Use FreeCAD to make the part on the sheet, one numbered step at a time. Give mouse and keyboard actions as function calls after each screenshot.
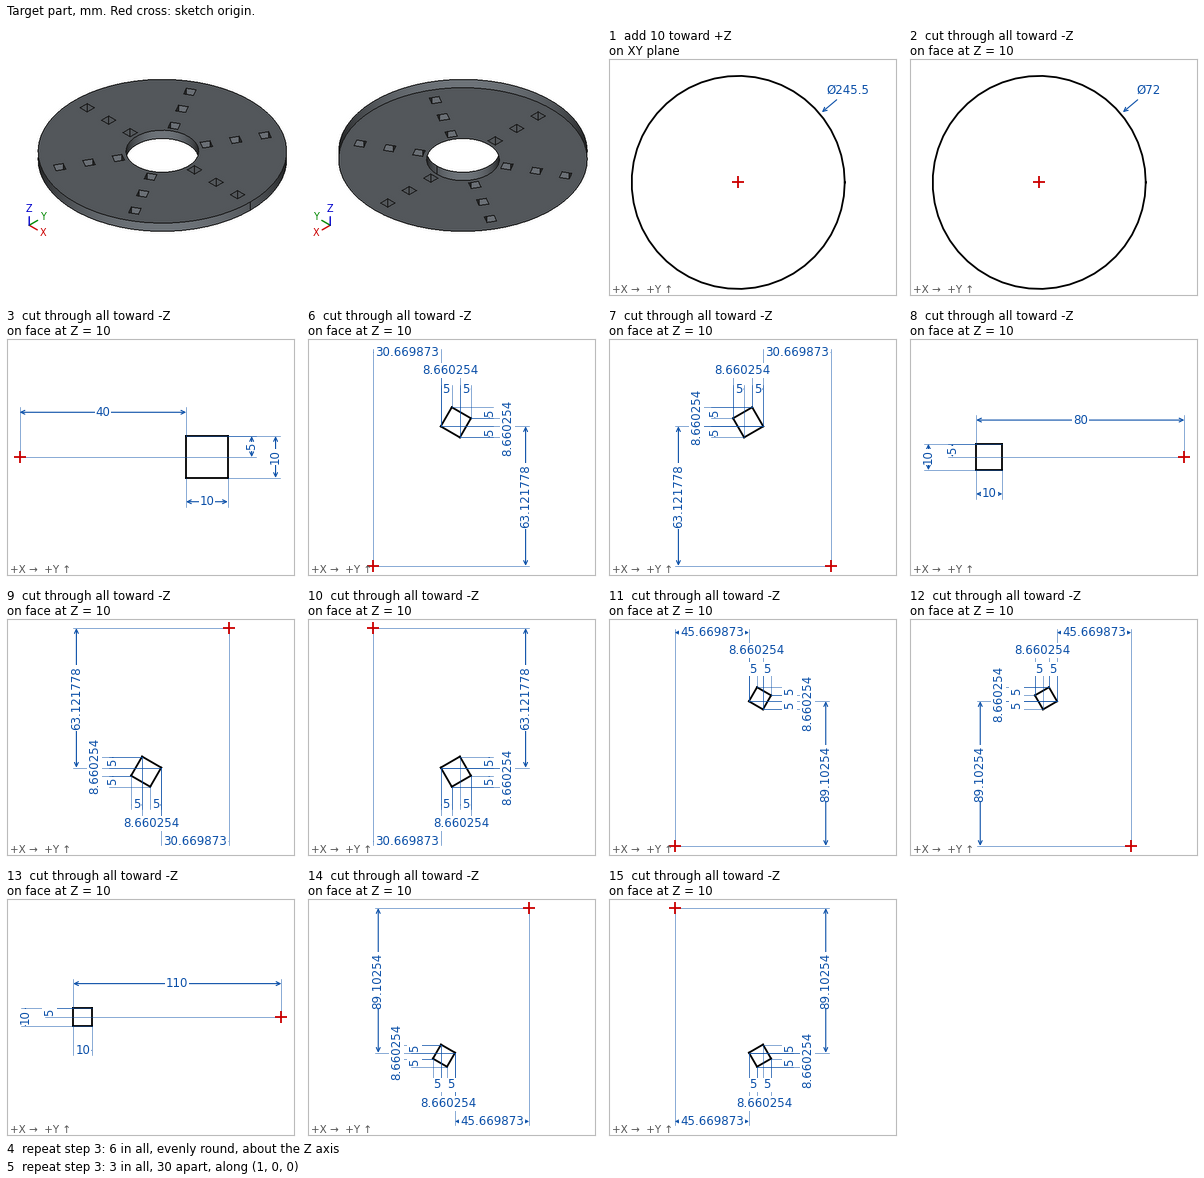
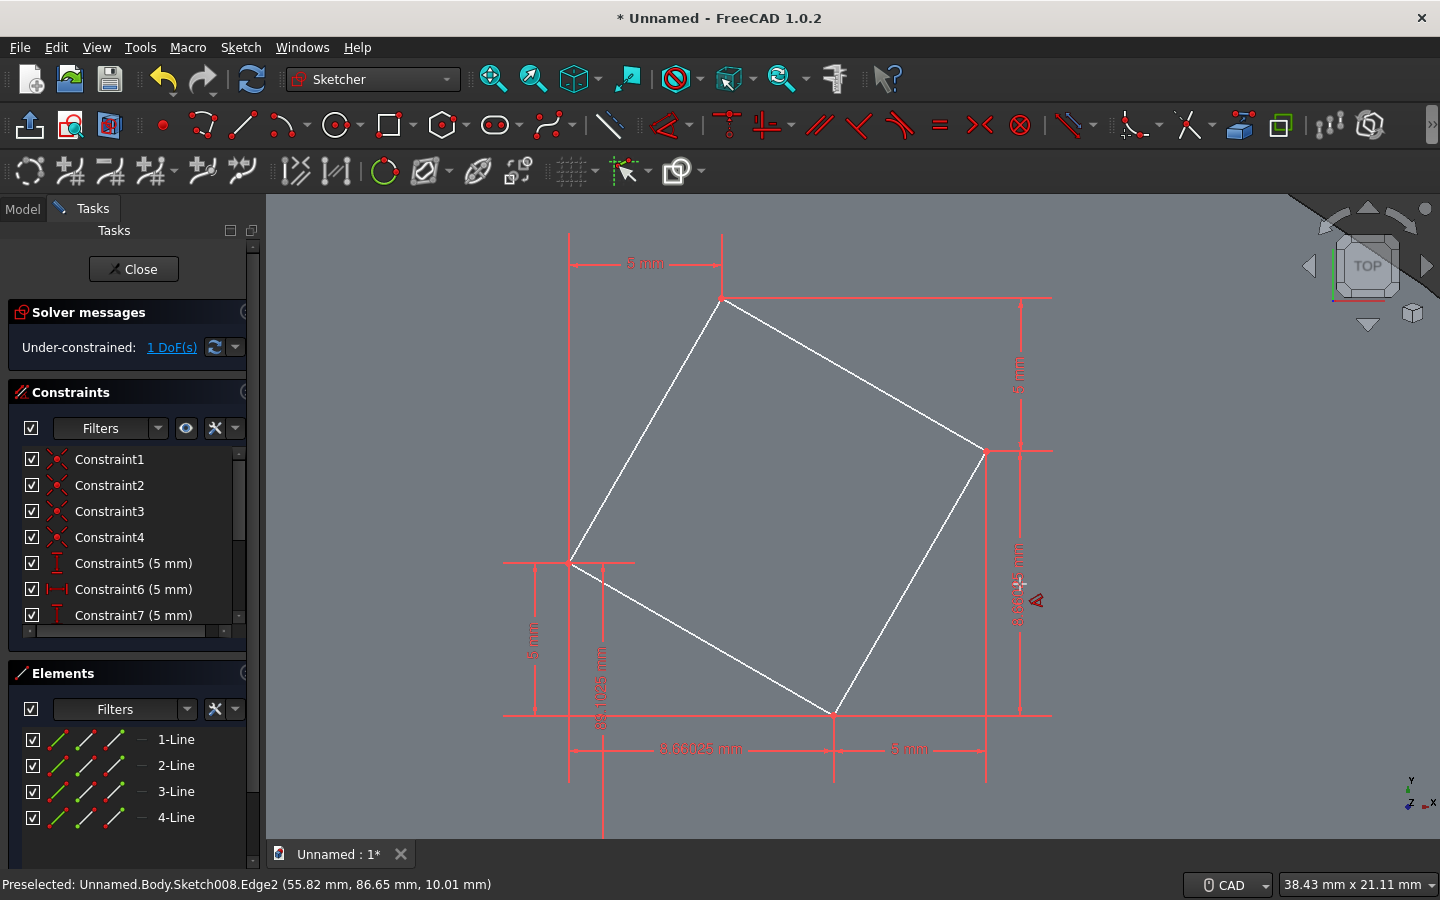
click(569, 563)
click(431, 529)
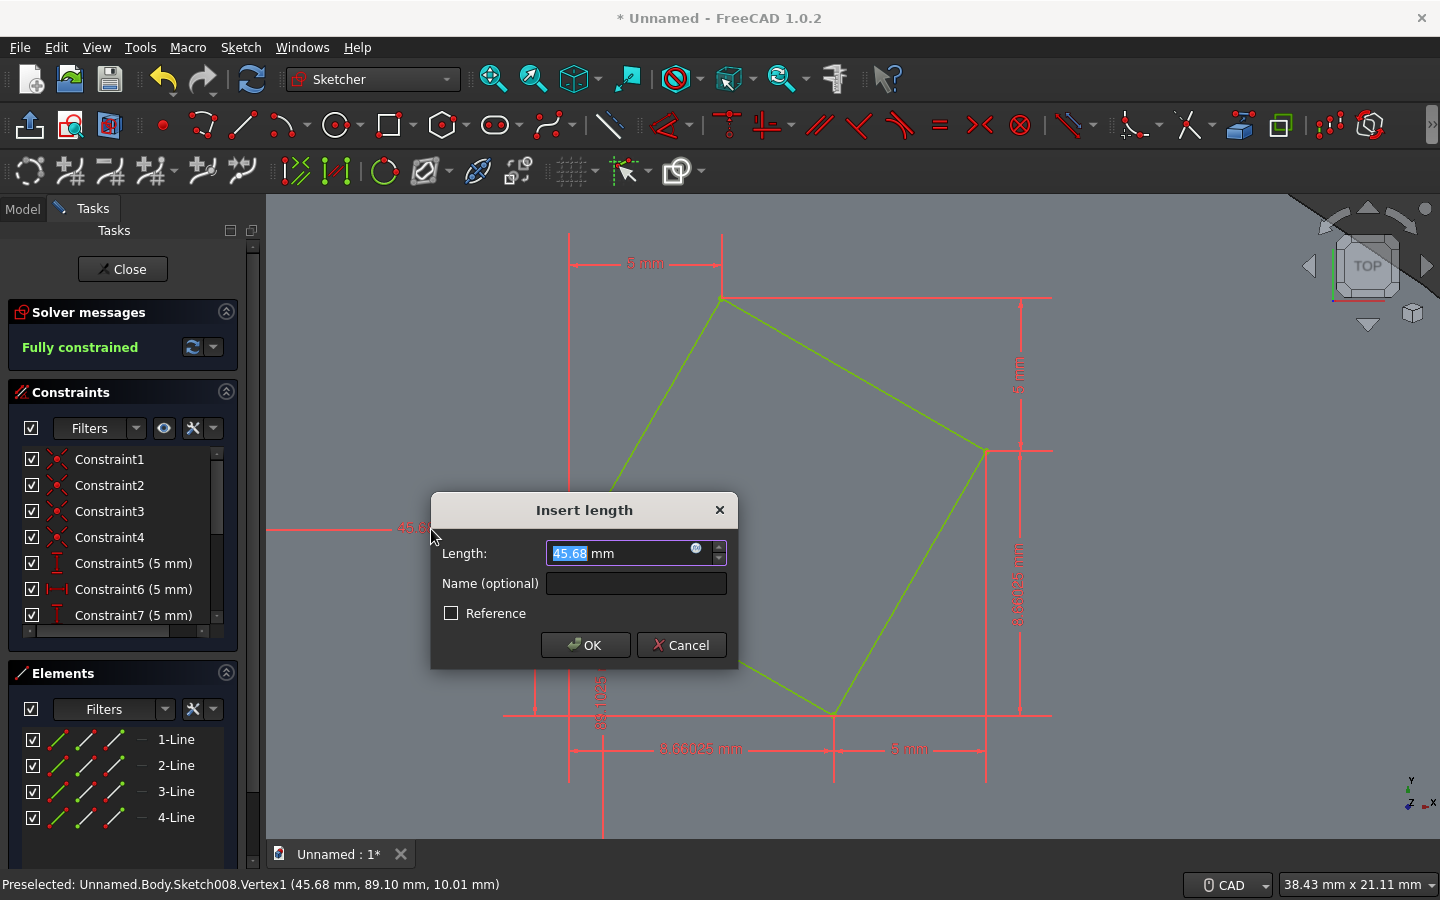
text(45.669873)
key(Return)
key(Escape)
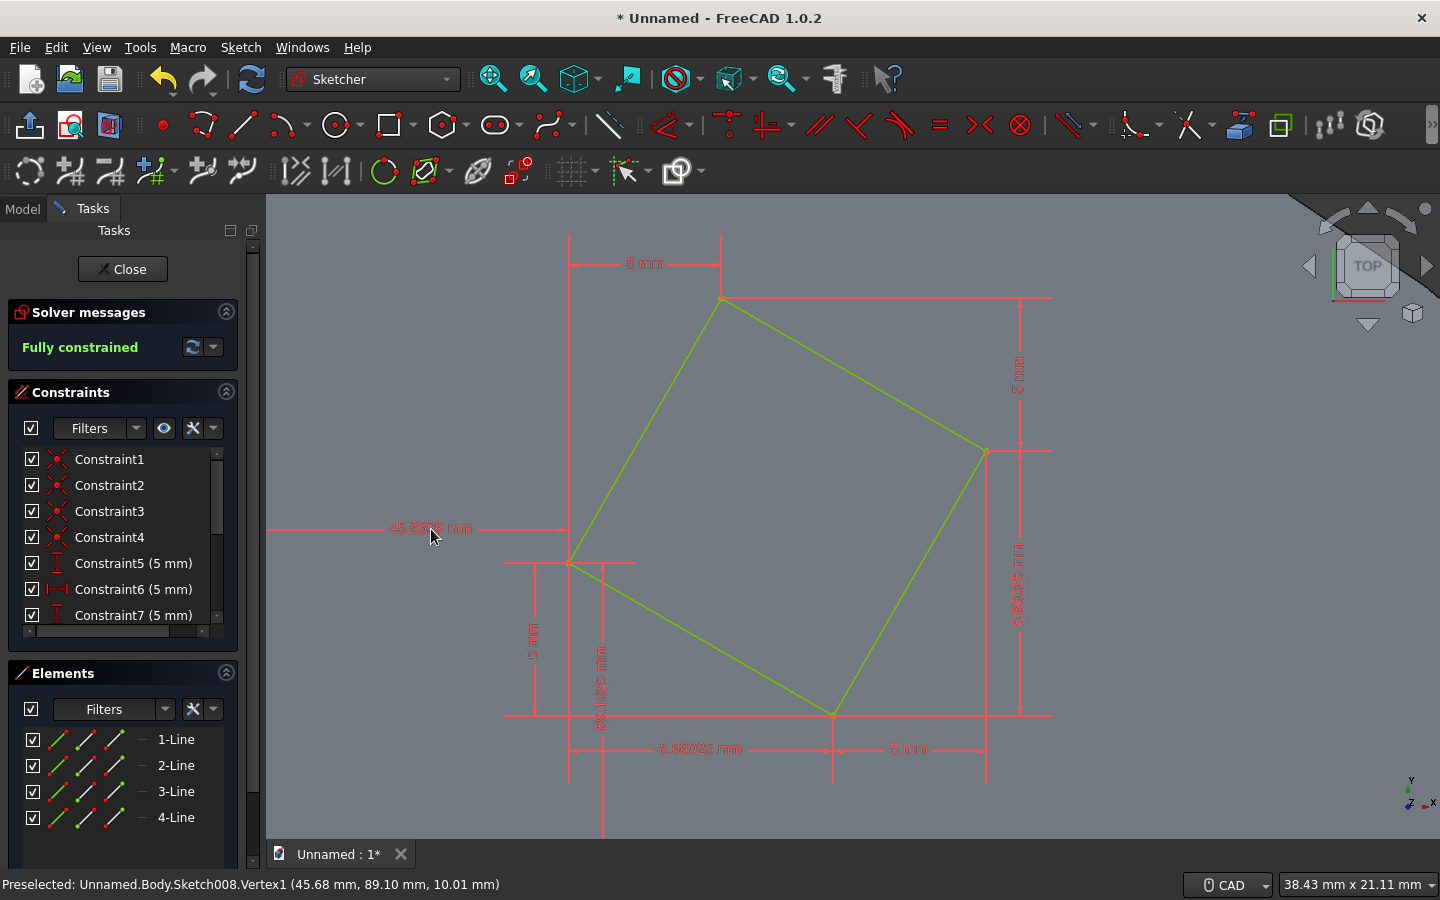
click(123, 269)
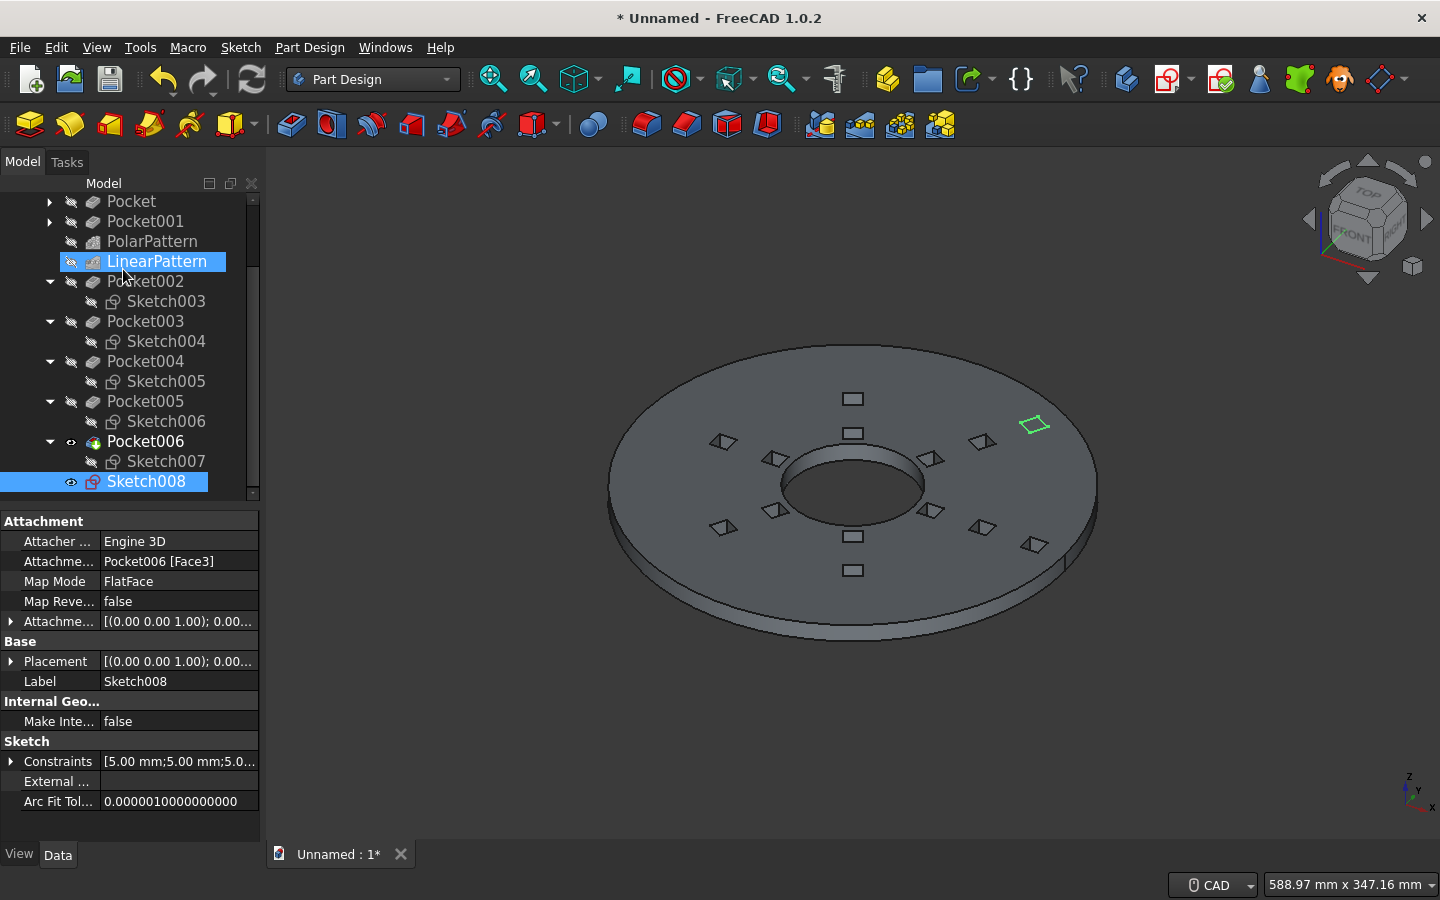
click(292, 124)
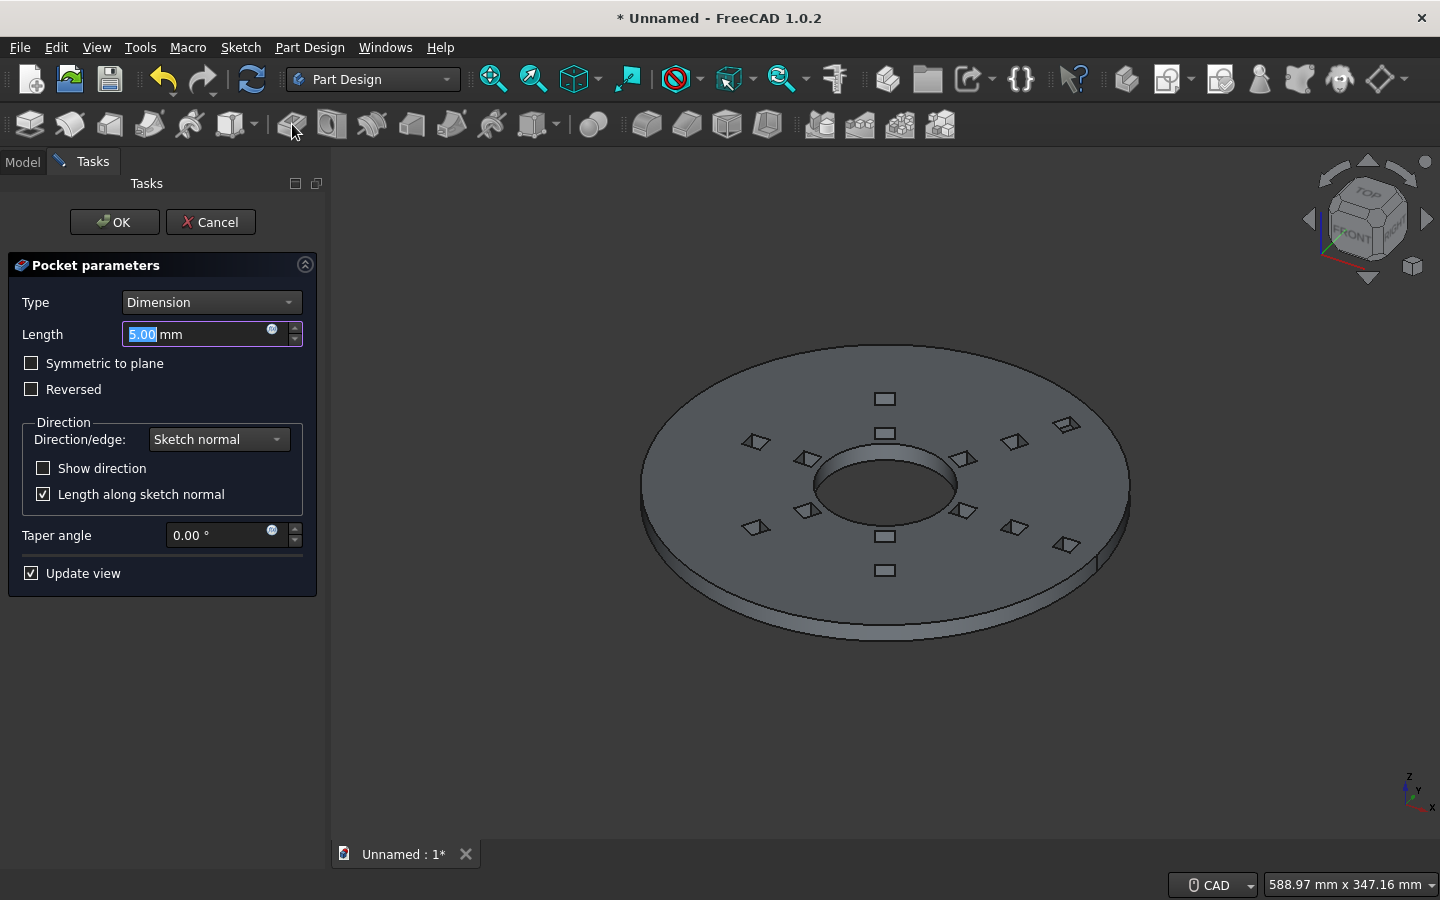
click(212, 302)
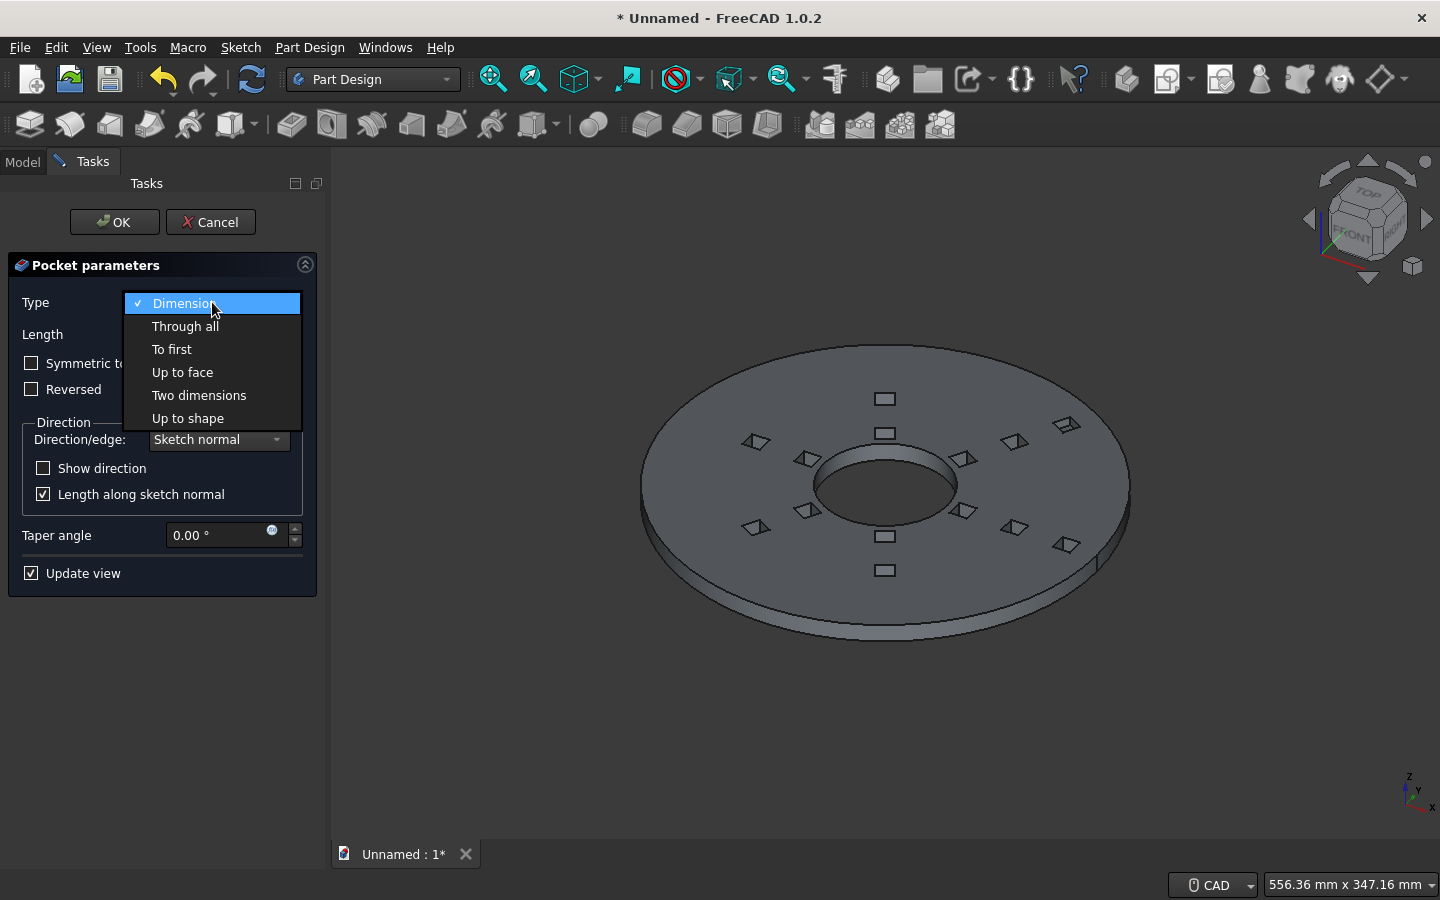
click(212, 326)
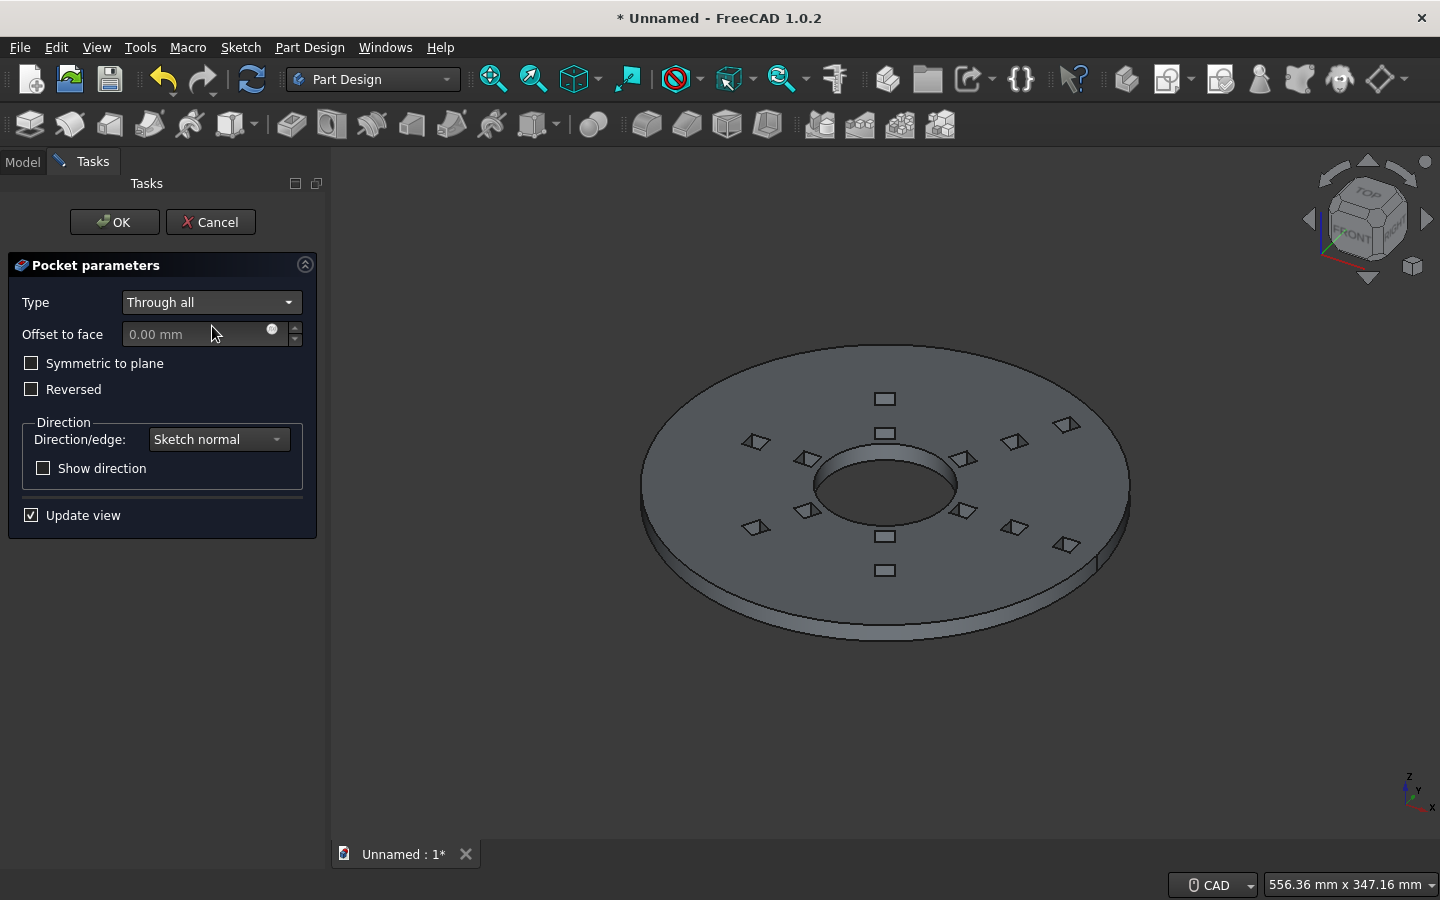
click(115, 222)